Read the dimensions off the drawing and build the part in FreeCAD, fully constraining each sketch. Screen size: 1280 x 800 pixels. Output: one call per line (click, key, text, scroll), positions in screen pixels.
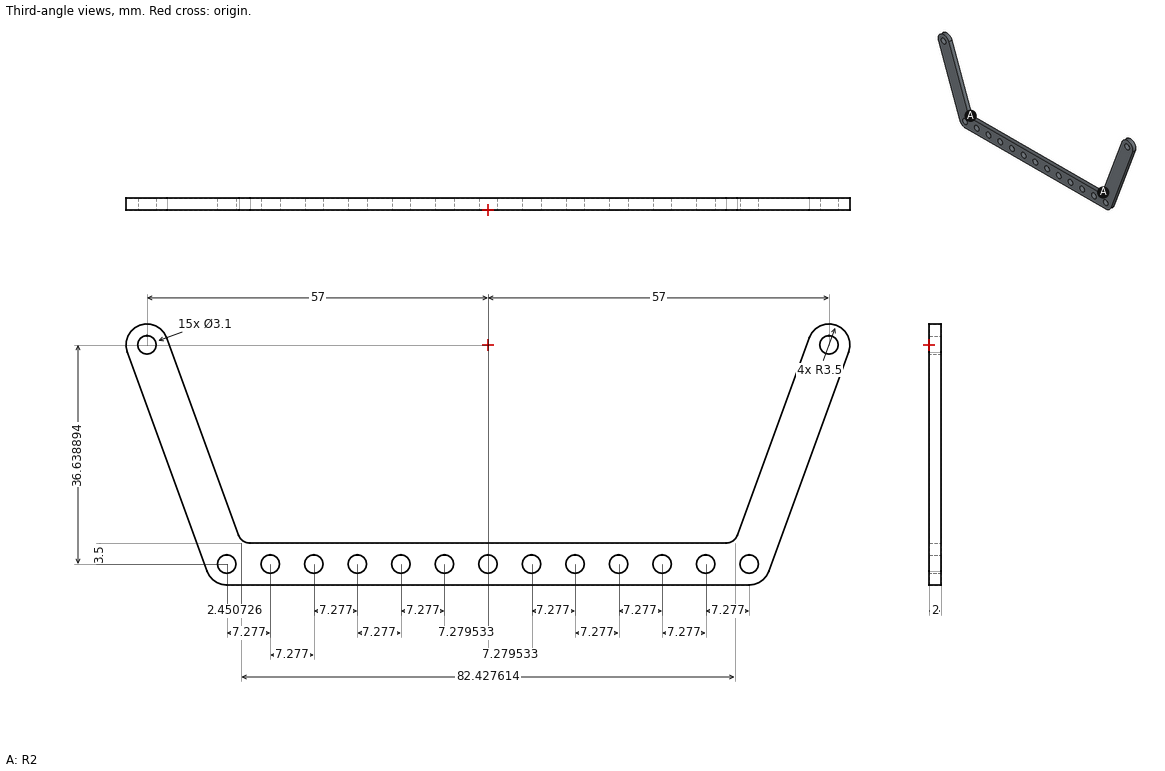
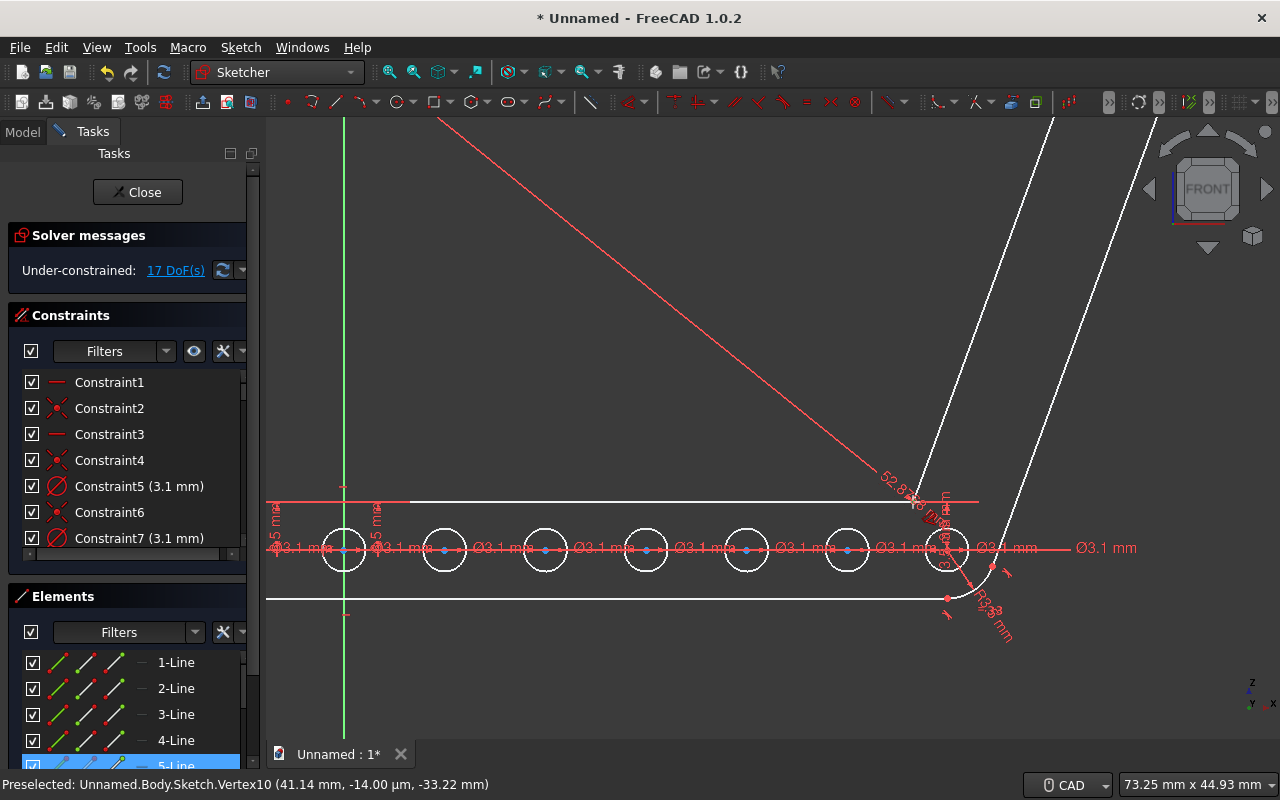
click(646, 550)
click(612, 526)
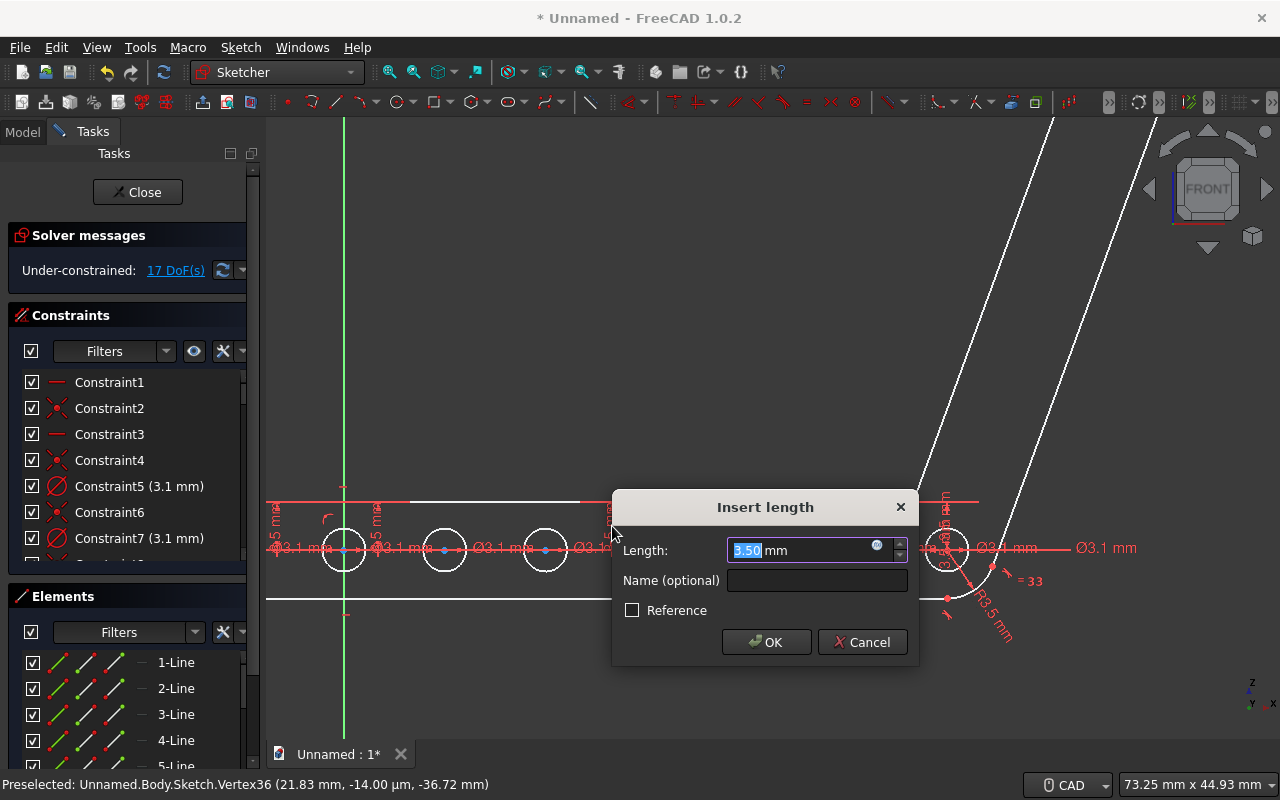
text(3.5)
key(Return)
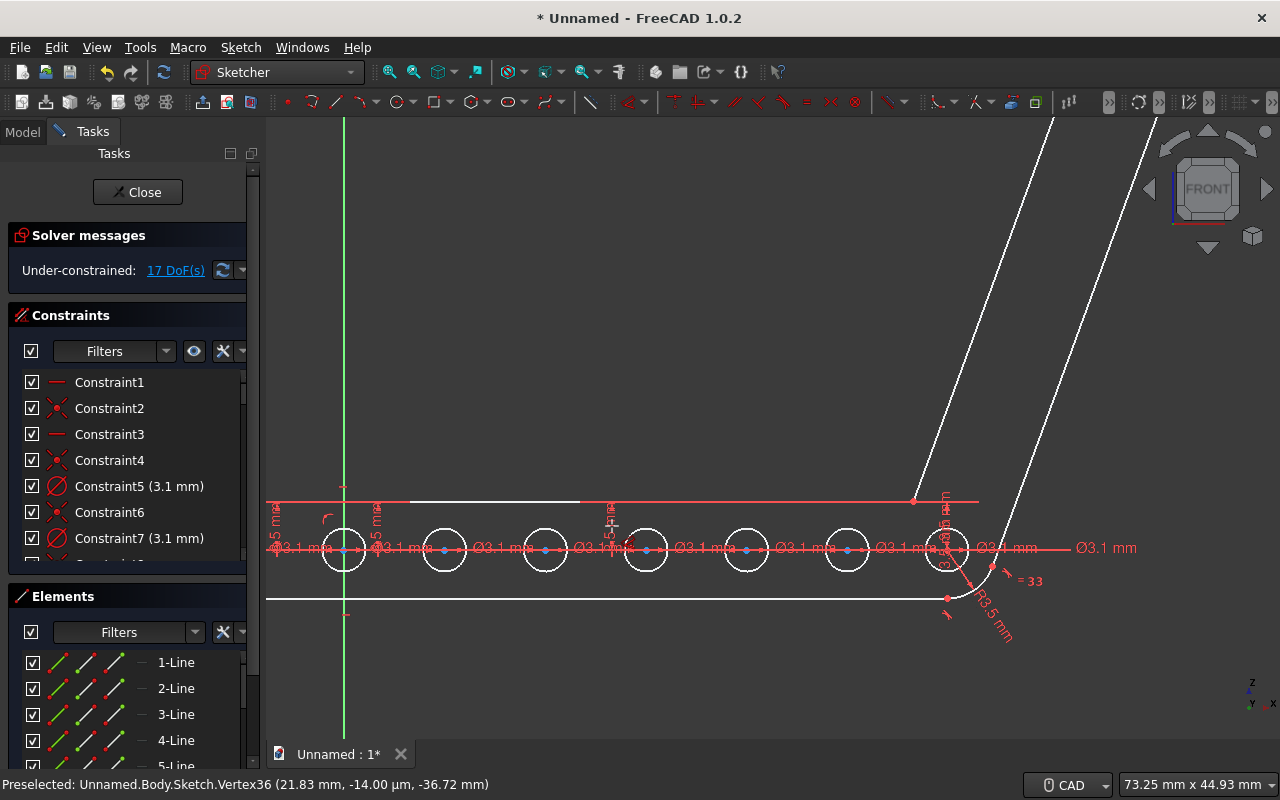
click(913, 502)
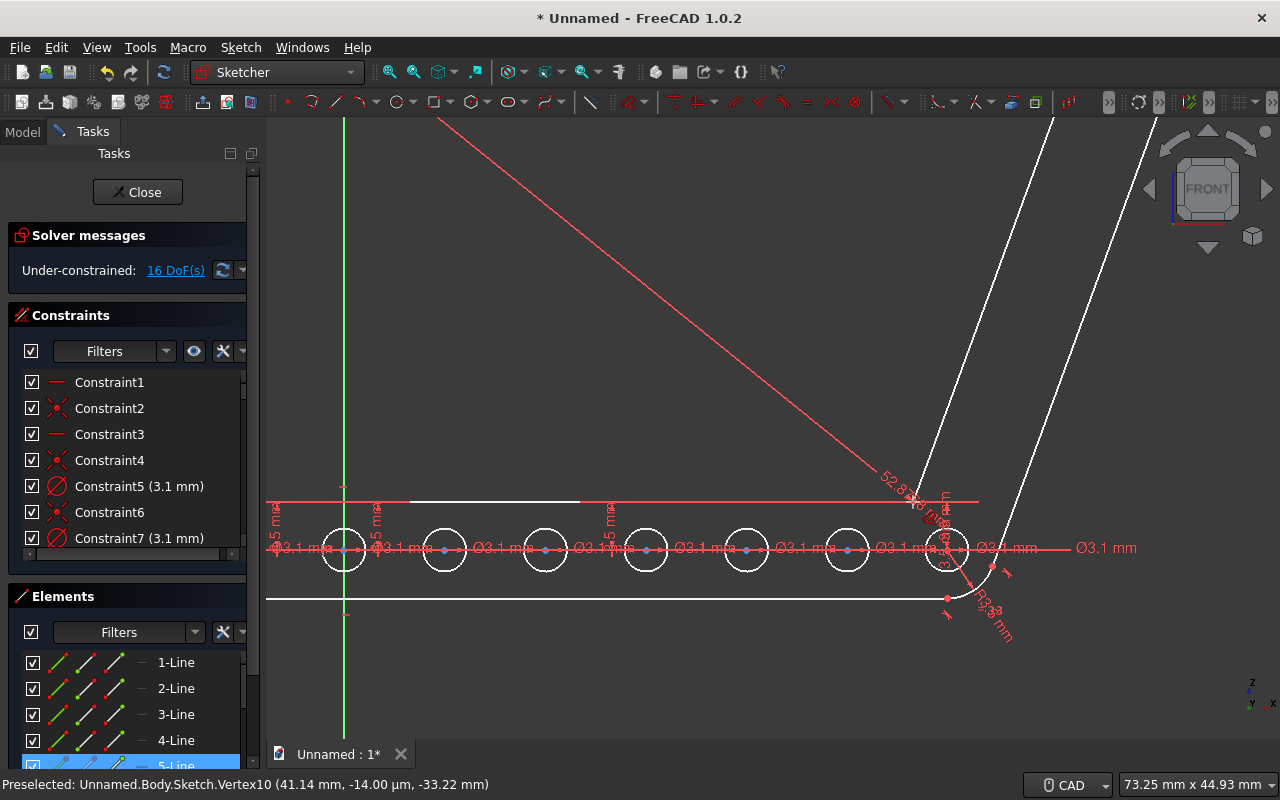
click(747, 550)
click(713, 526)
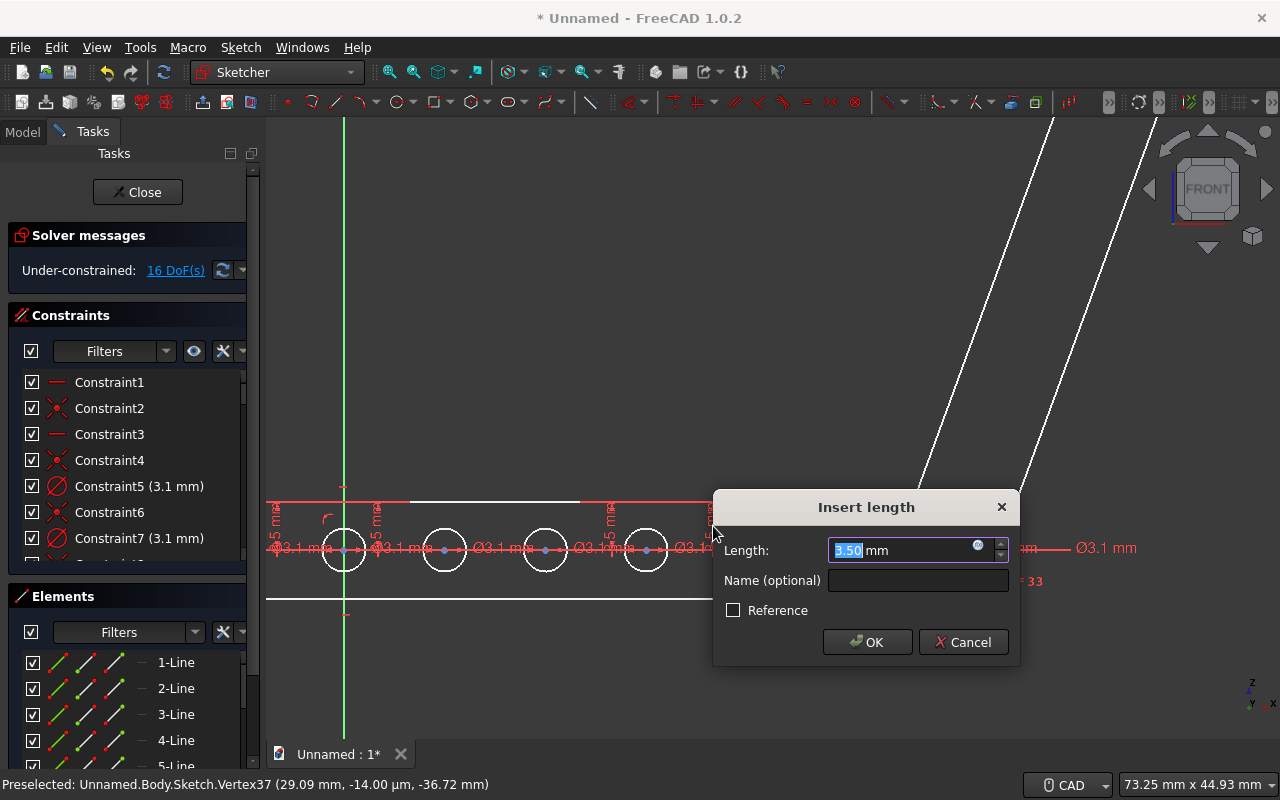
text(3.5)
key(Return)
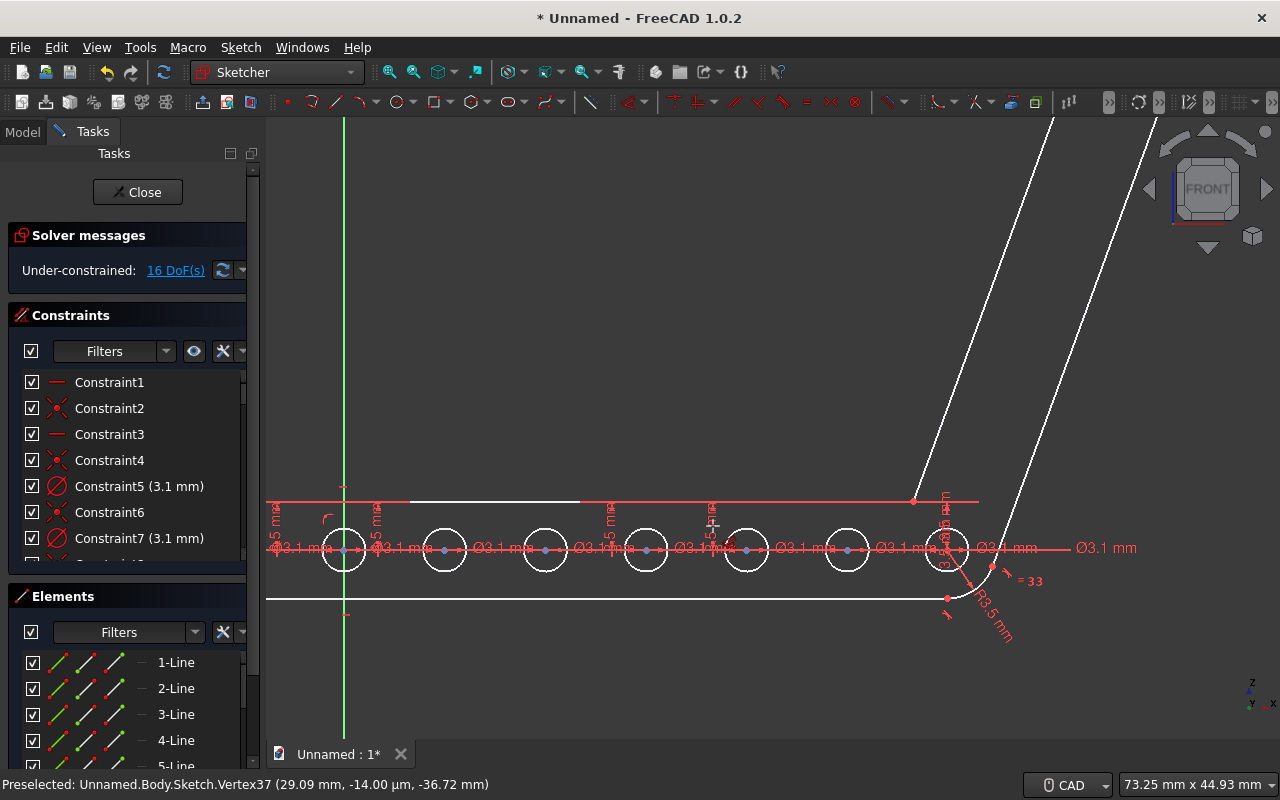
click(913, 502)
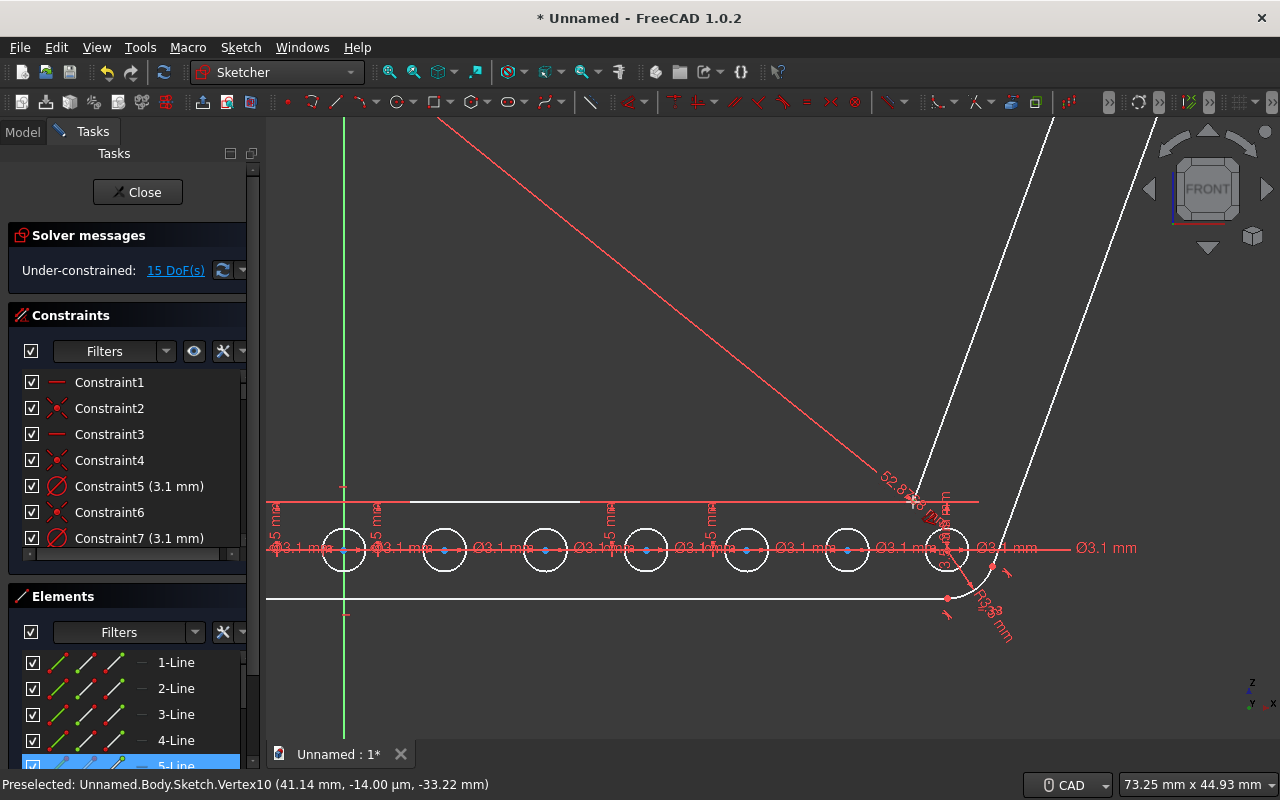
click(847, 550)
click(813, 526)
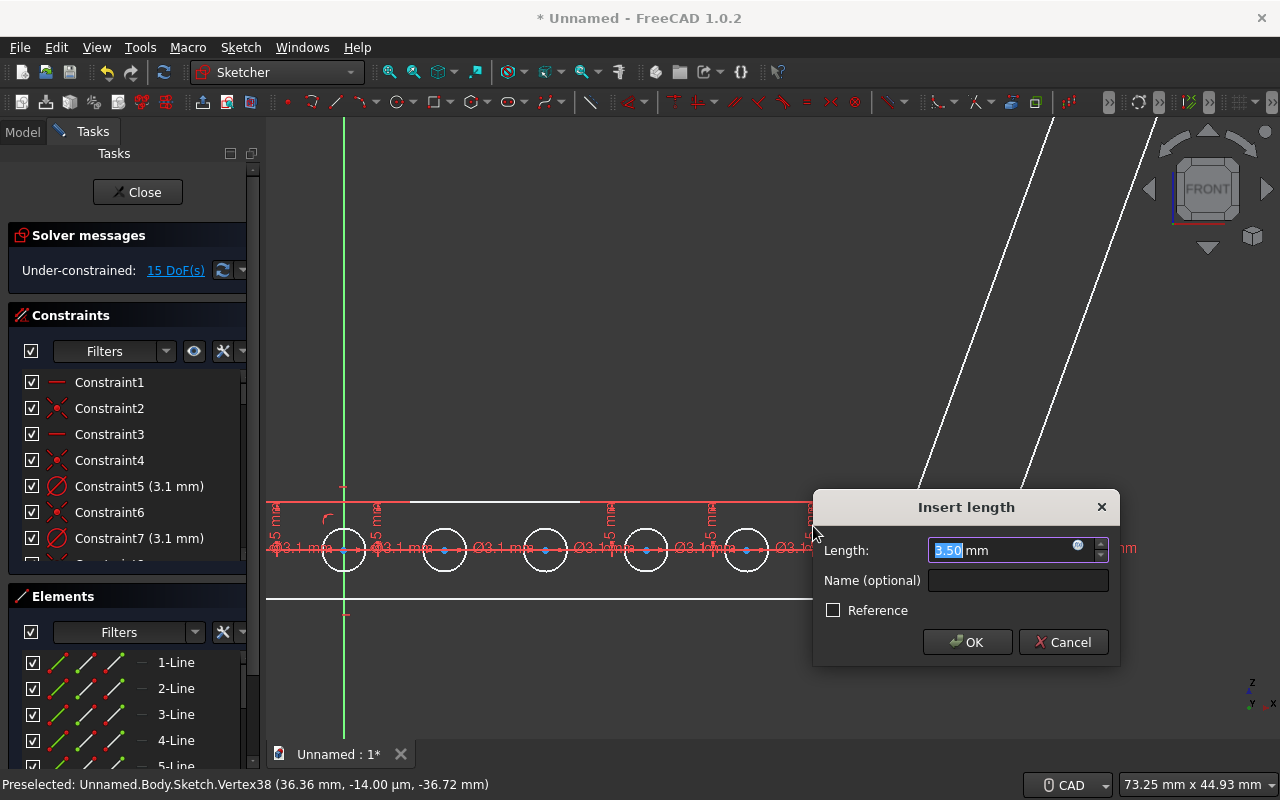
text(3.5)
key(Return)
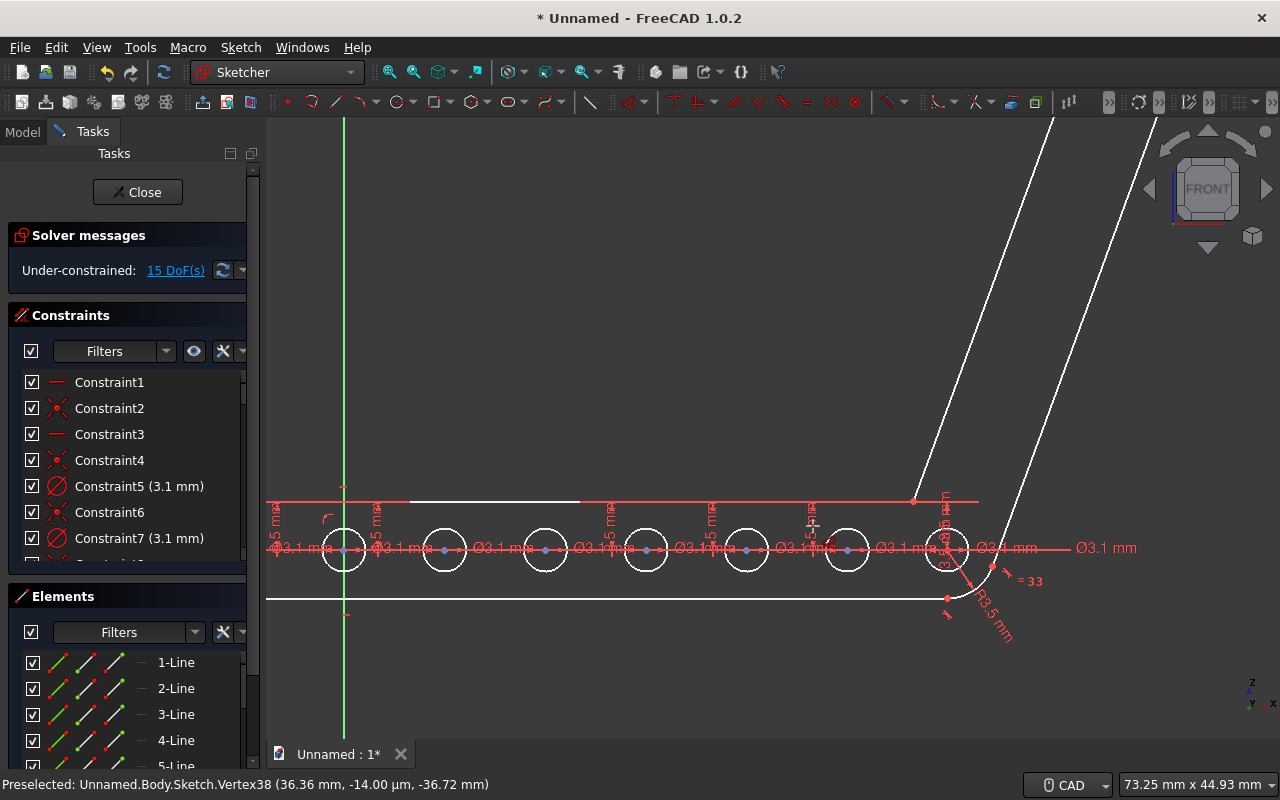
scroll(914, 504, down, 5)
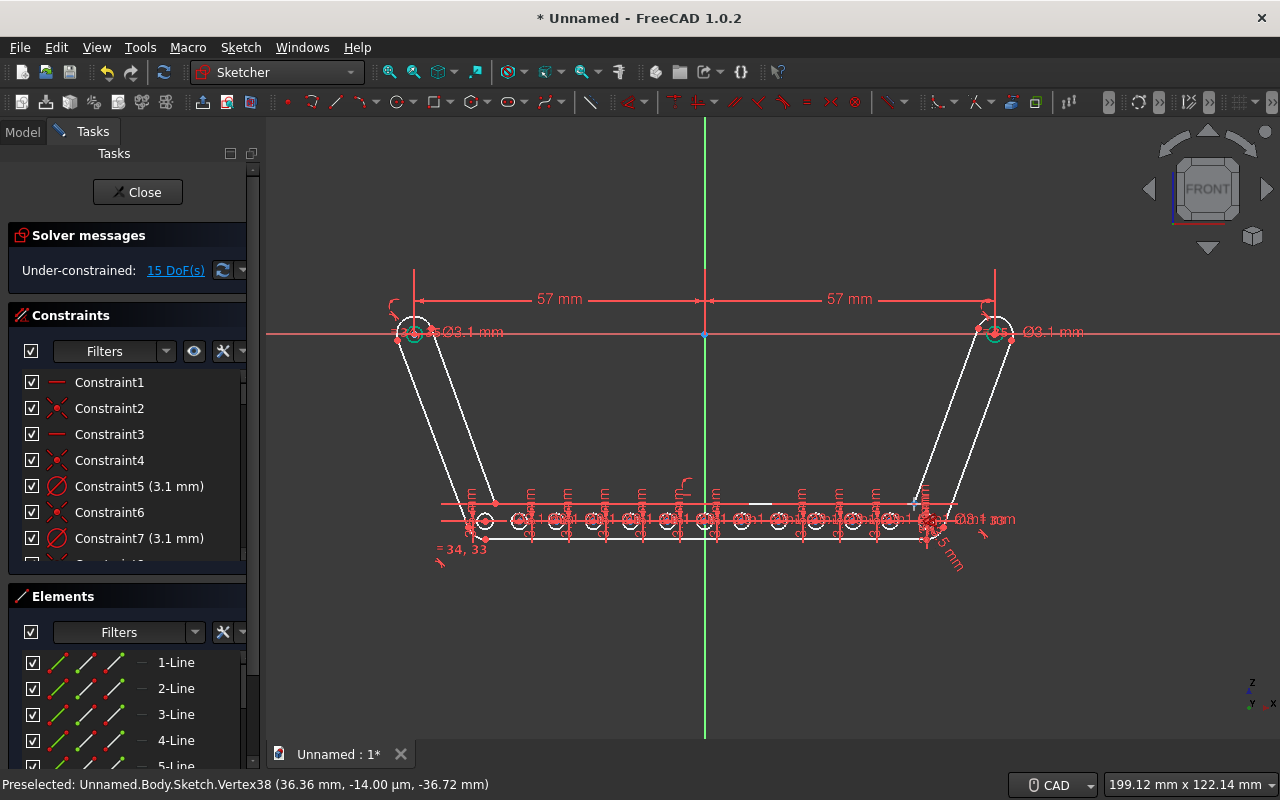
click(485, 521)